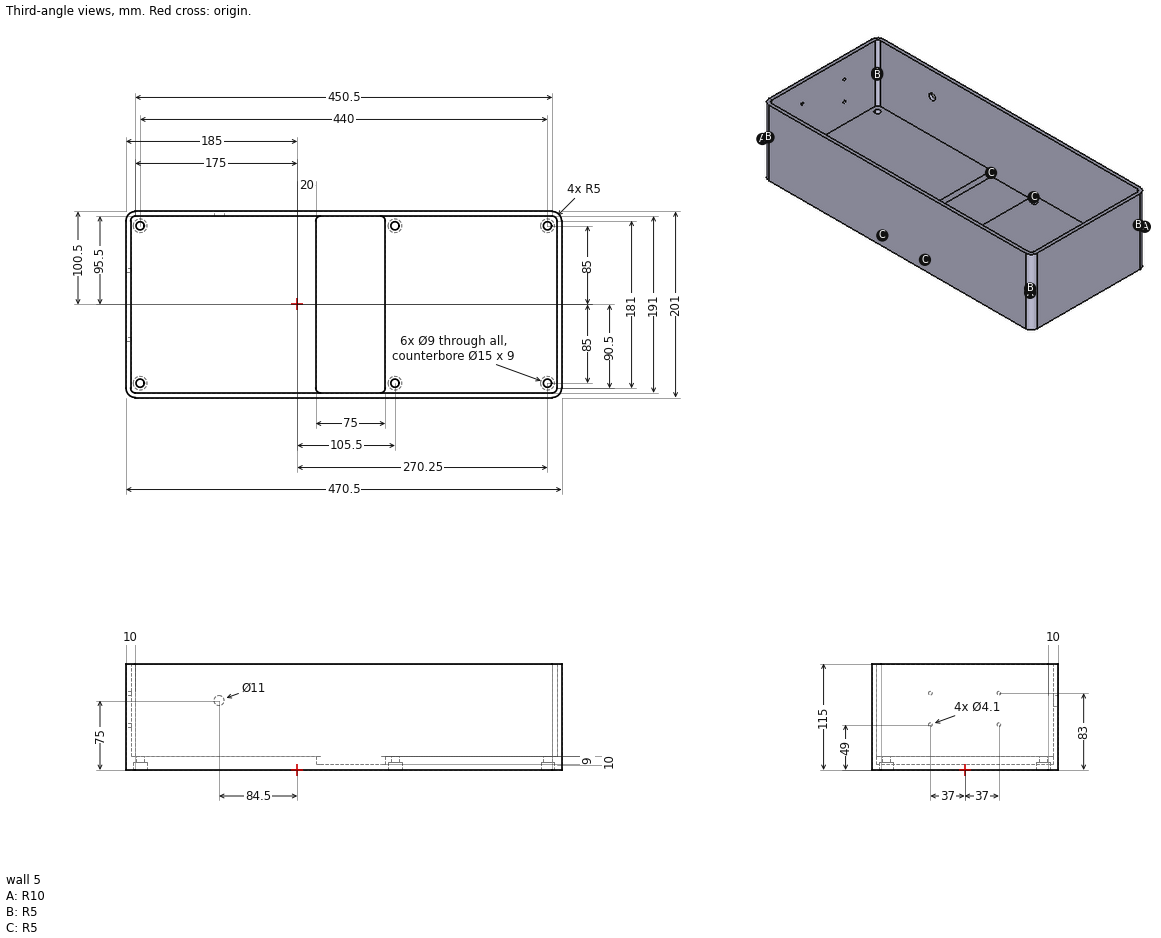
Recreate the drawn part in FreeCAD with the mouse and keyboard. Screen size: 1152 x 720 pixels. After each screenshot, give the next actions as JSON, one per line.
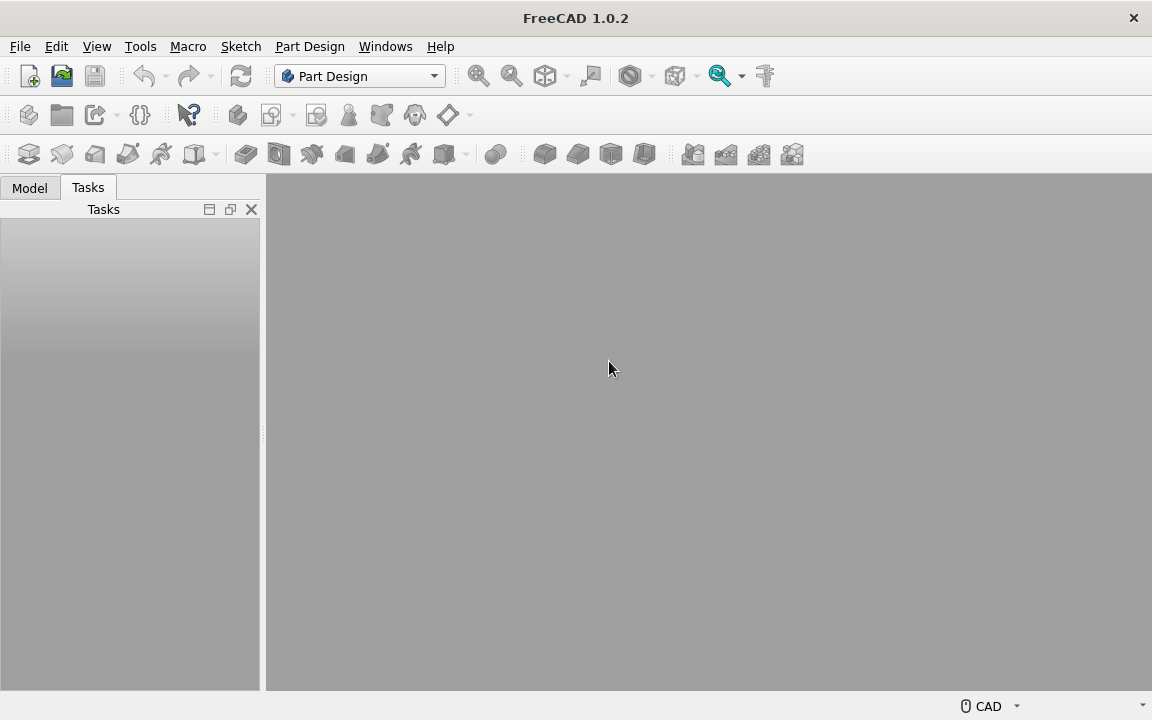
{"action": "left_click", "coordinate": [29, 76]}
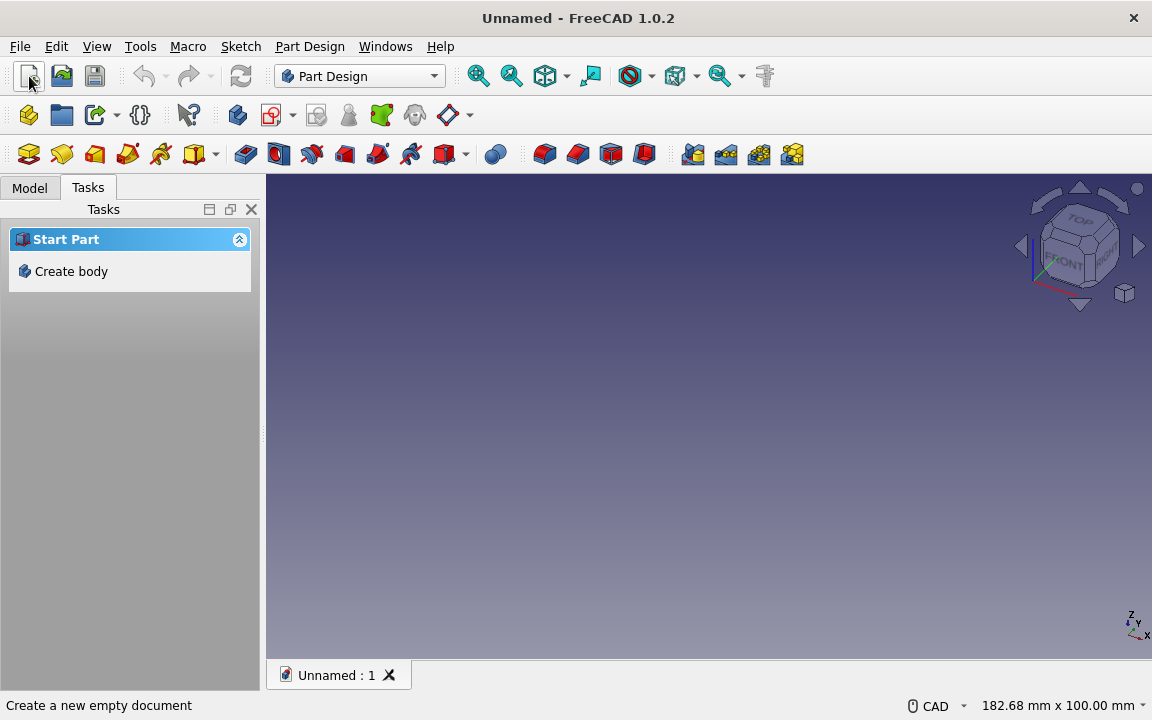
{"action": "left_click", "coordinate": [270, 116]}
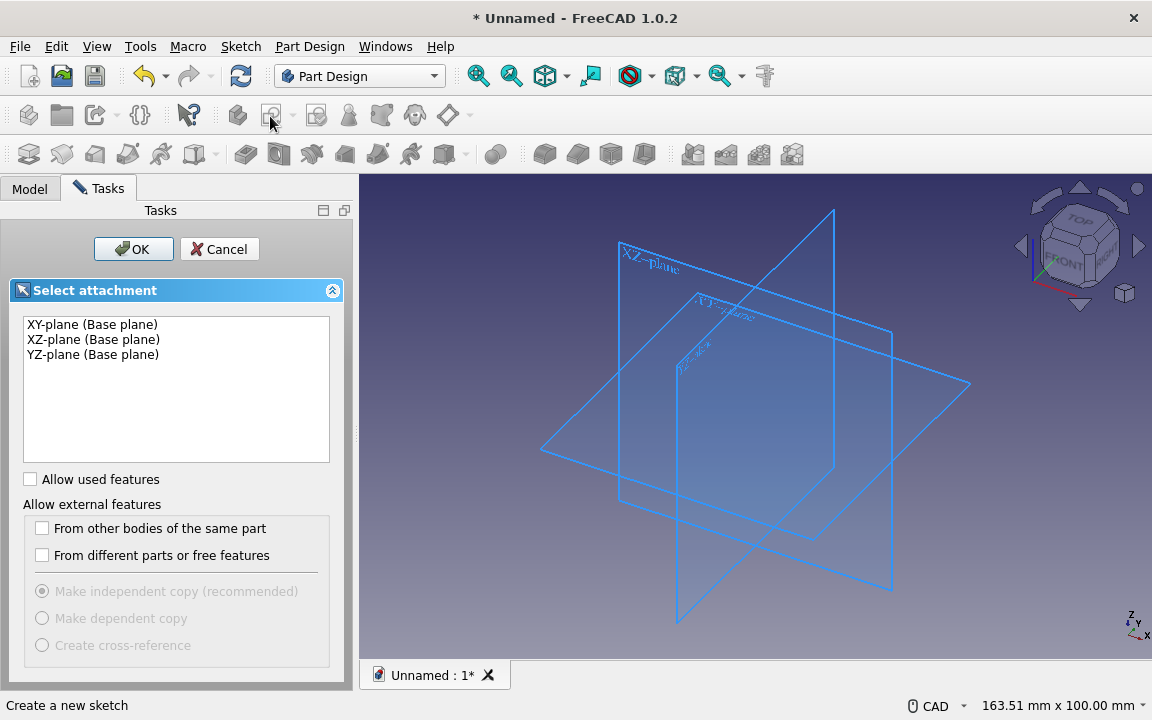
{"action": "left_click", "coordinate": [84, 324]}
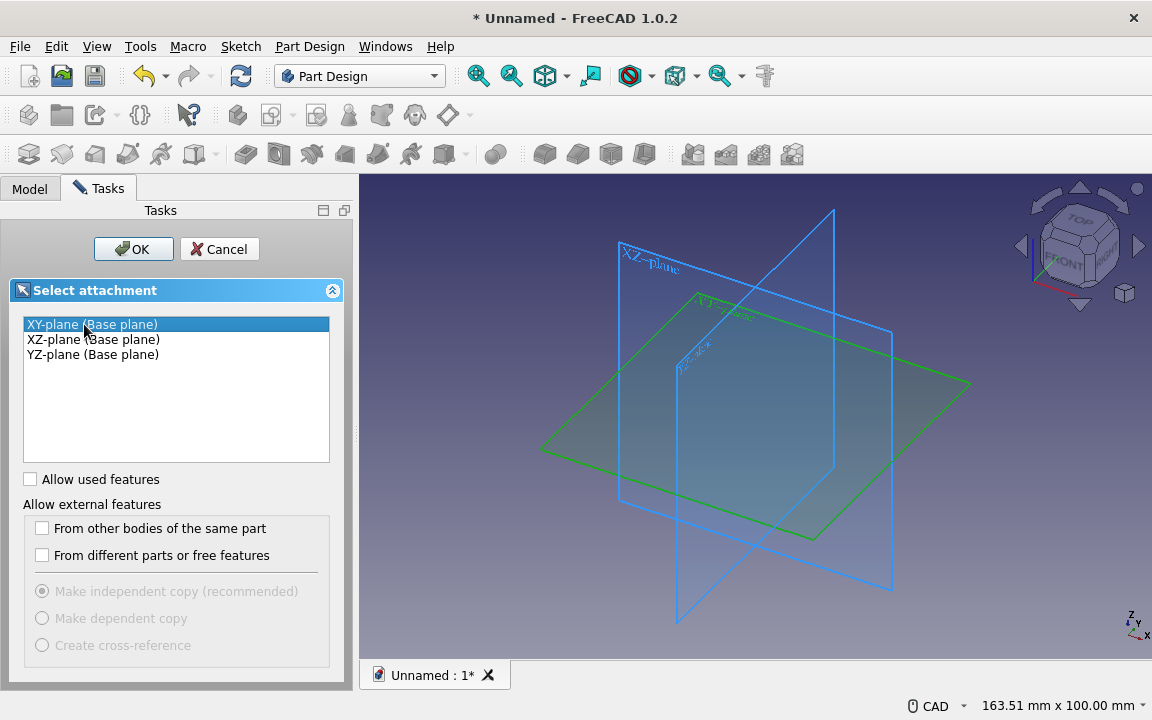
{"action": "left_click", "coordinate": [134, 249]}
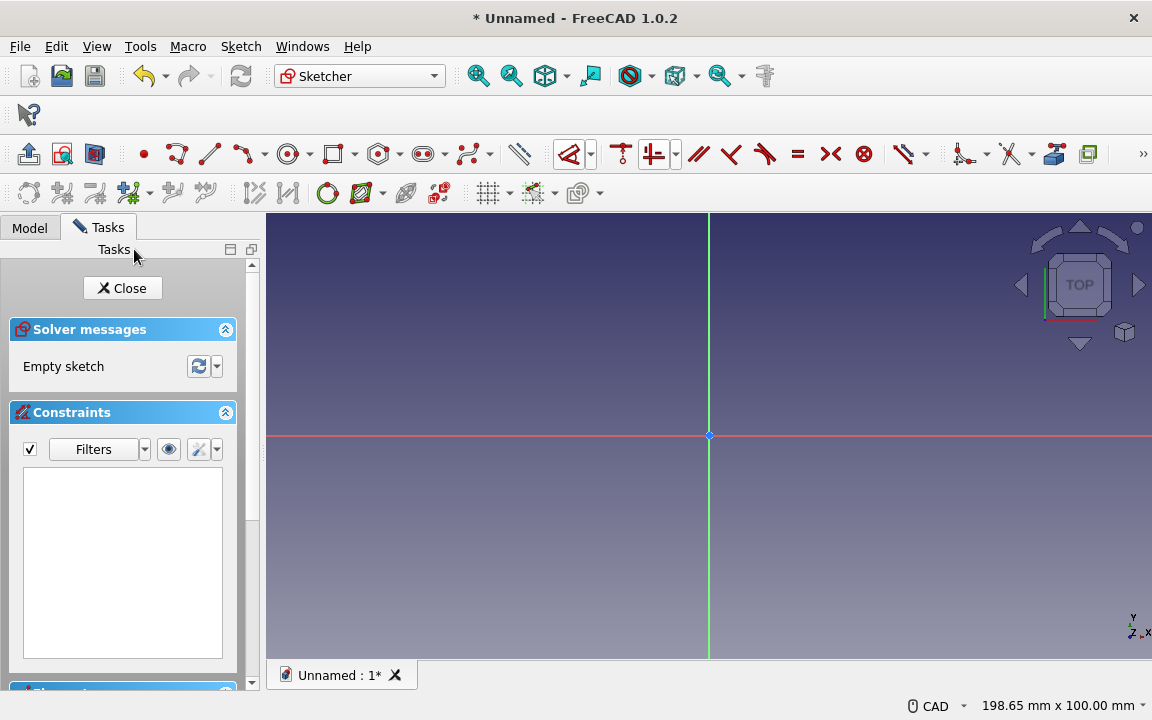
{"action": "scroll", "coordinate": [545, 436], "scroll_direction": "down", "scroll_amount": 7}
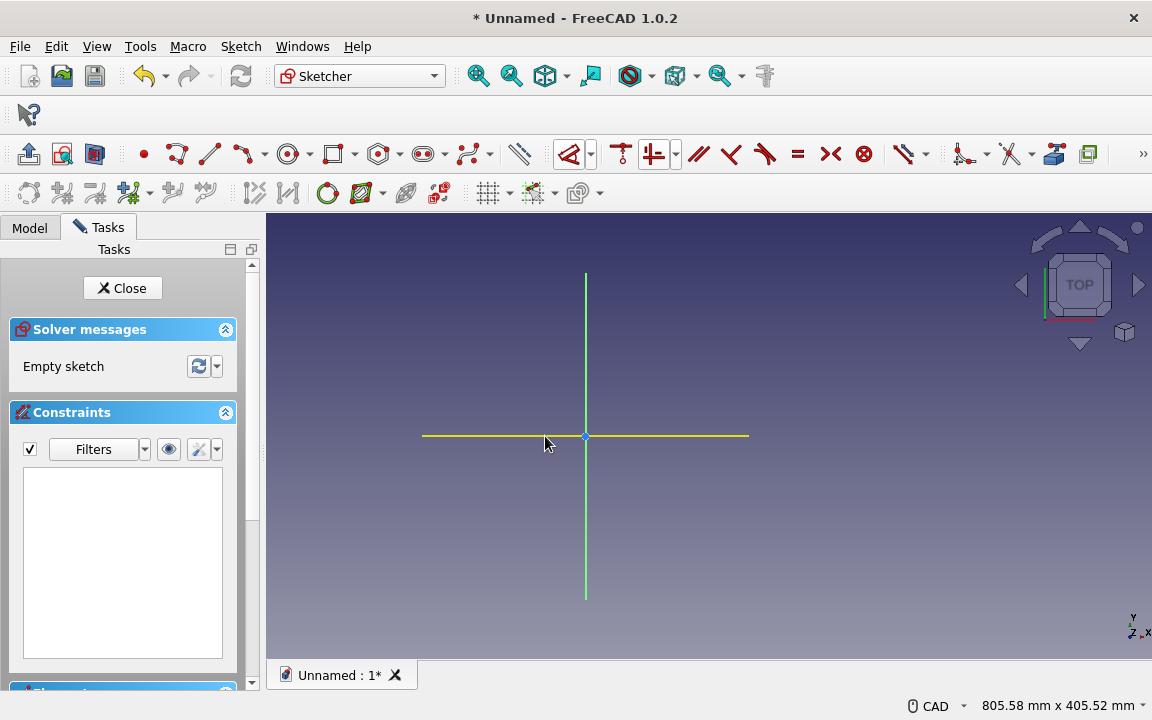
{"action": "key", "text": "g r"}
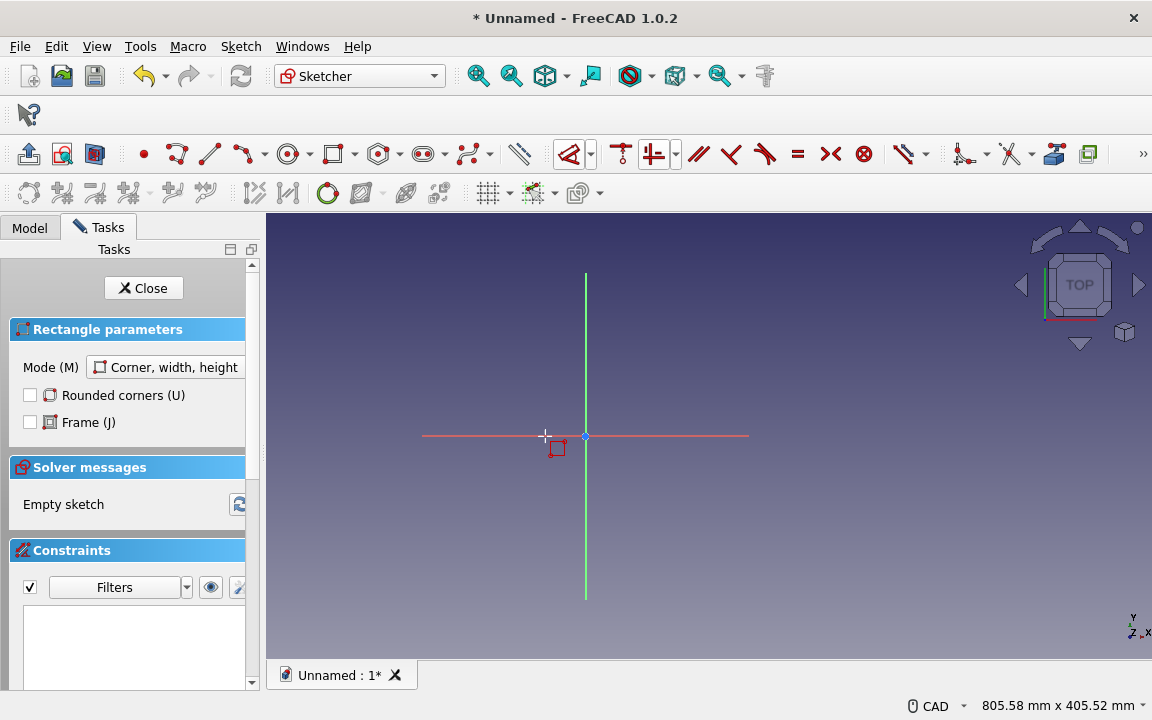
{"action": "left_click", "coordinate": [382, 326]}
{"action": "mouse_move", "coordinate": [900, 547]}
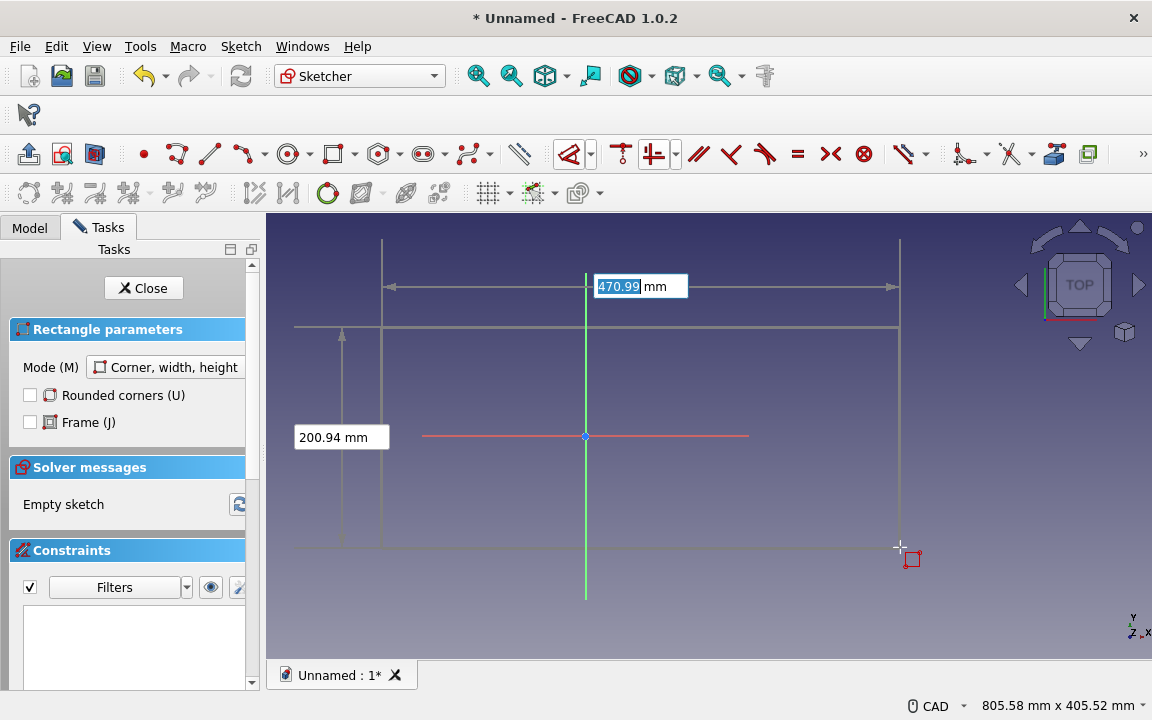
{"action": "type", "text": "470.5"}
{"action": "key", "text": "Tab"}
{"action": "type", "text": "201"}
{"action": "key", "text": "Return"}
{"action": "key", "text": "Escape"}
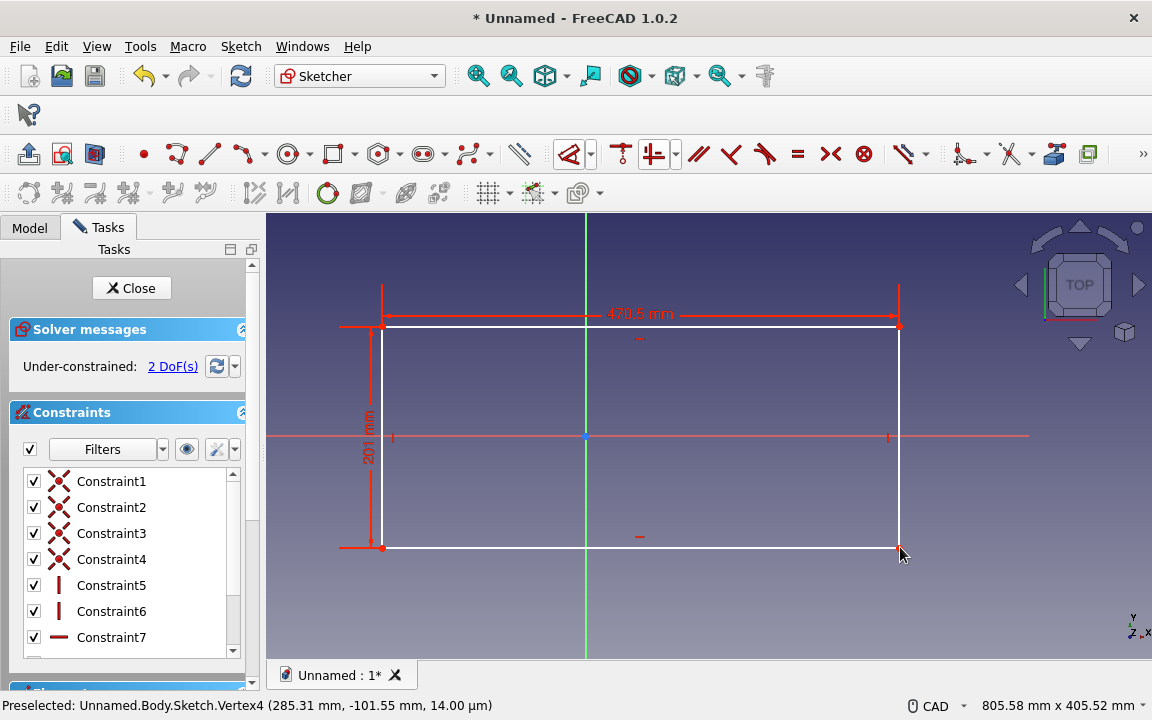
{"action": "key", "text": "d"}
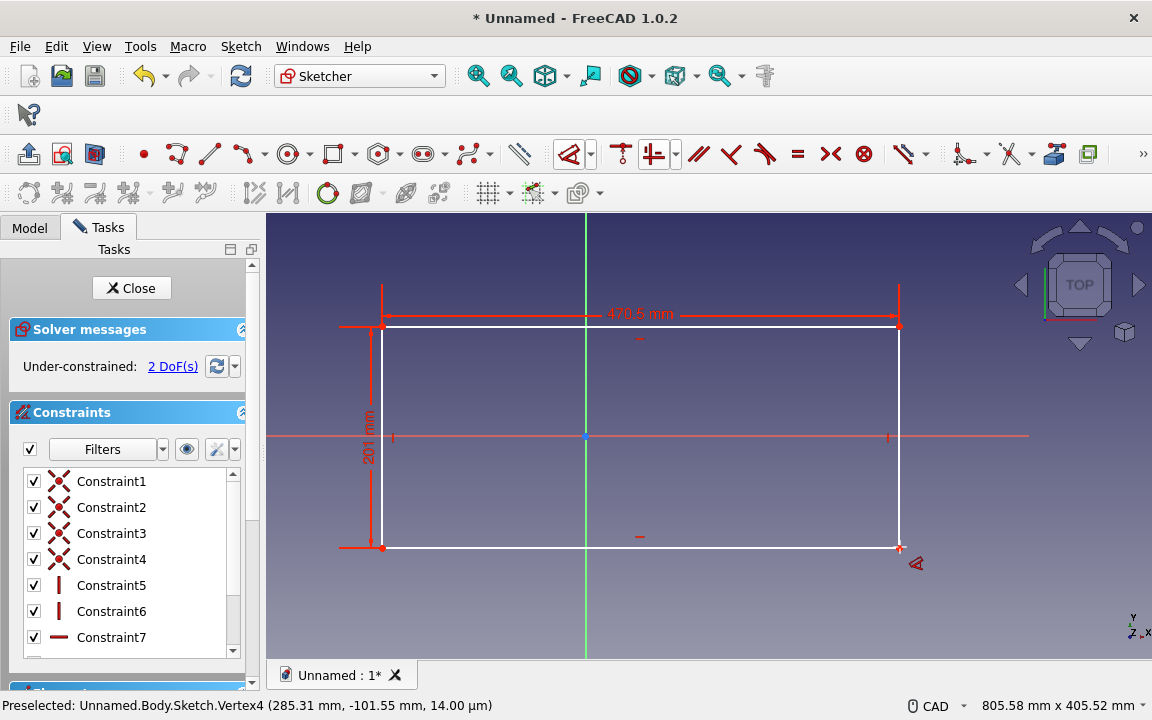
{"action": "left_click", "coordinate": [382, 327]}
{"action": "left_click", "coordinate": [484, 293]}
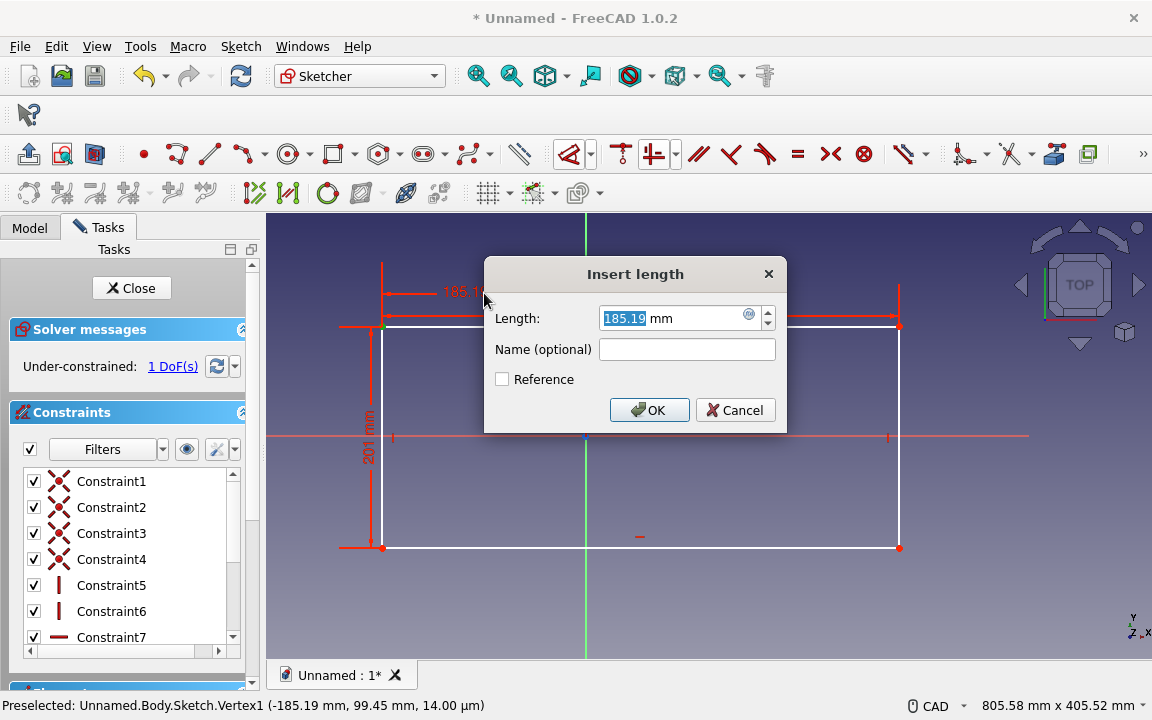
{"action": "type", "text": "185"}
{"action": "key", "text": "Return"}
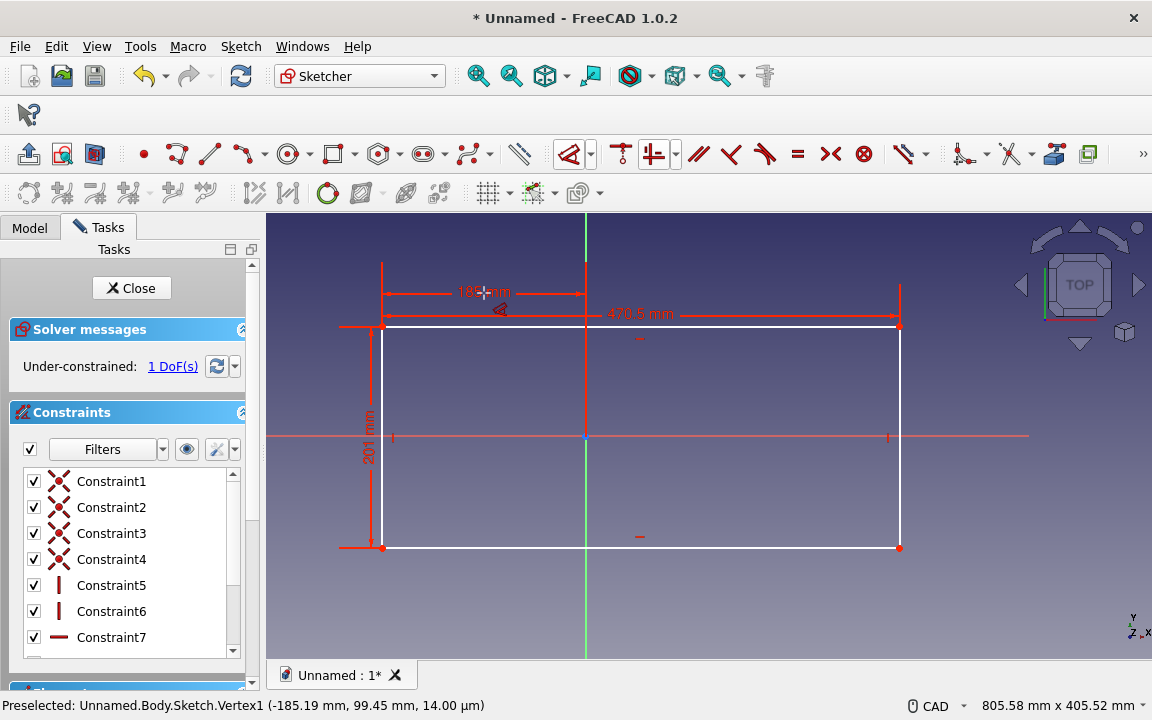
{"action": "left_click", "coordinate": [382, 327]}
{"action": "left_click", "coordinate": [348, 382]}